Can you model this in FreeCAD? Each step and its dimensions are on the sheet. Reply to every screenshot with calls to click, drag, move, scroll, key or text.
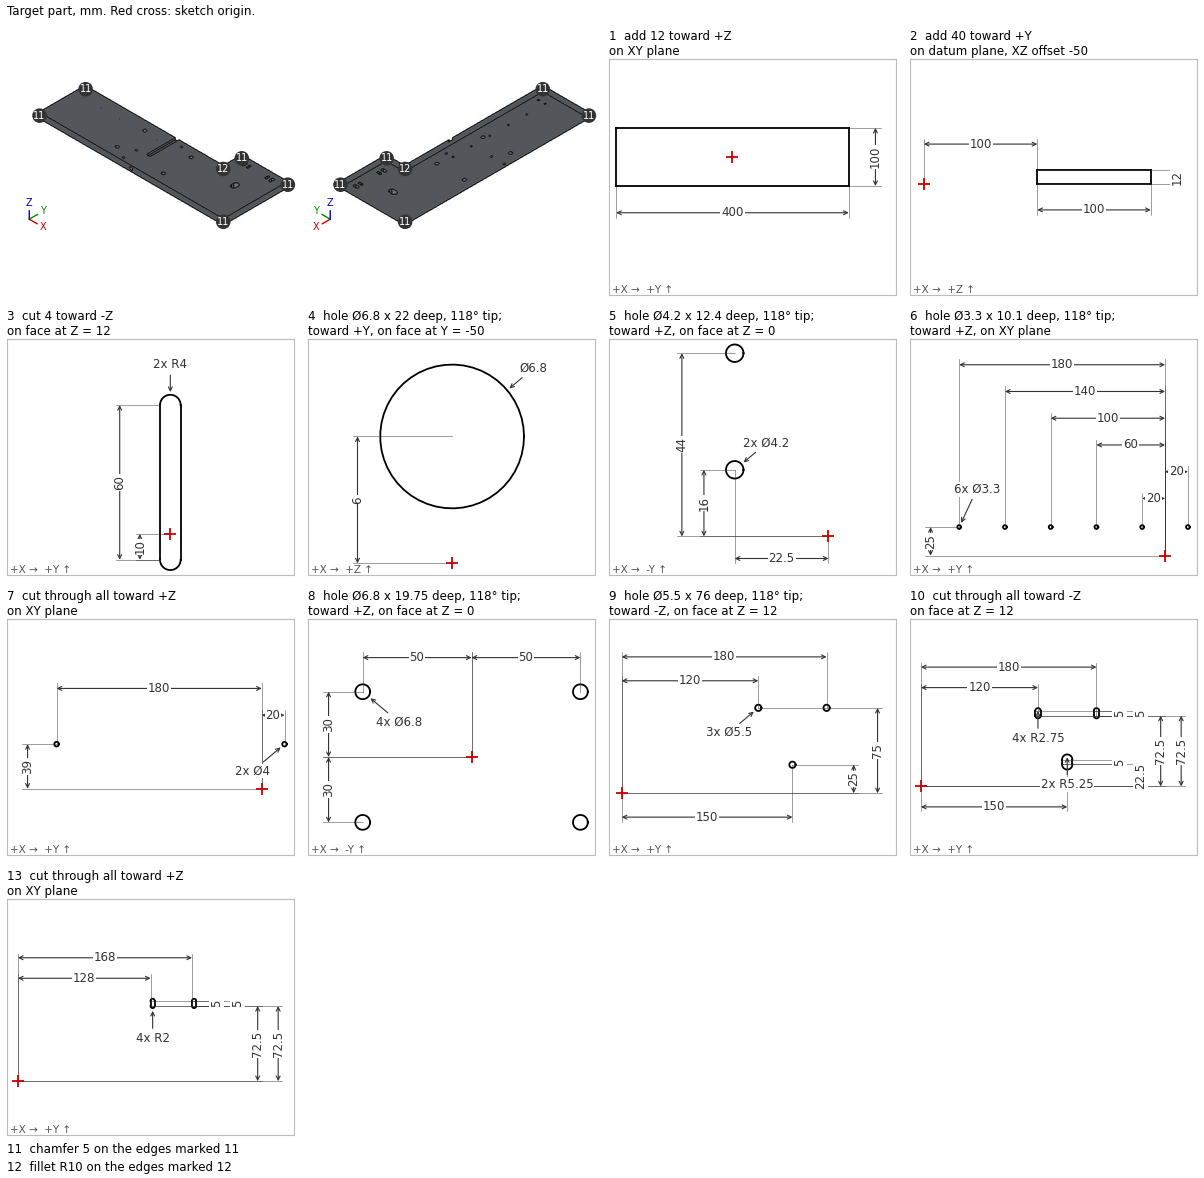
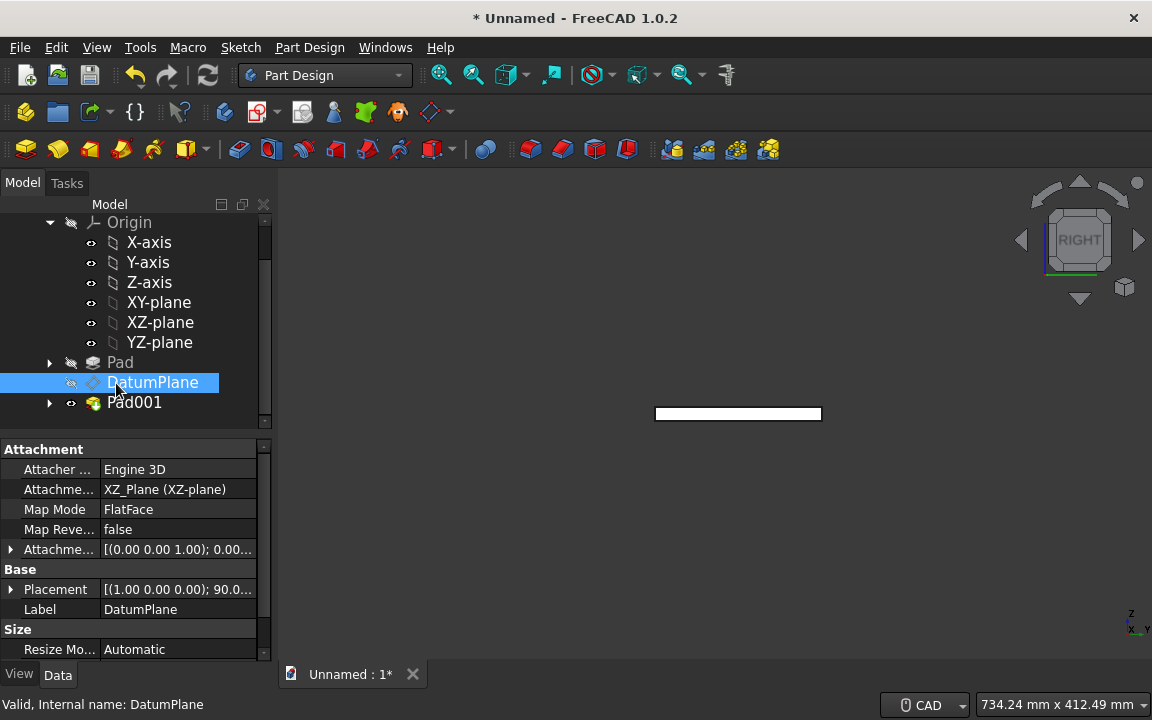
click(442, 76)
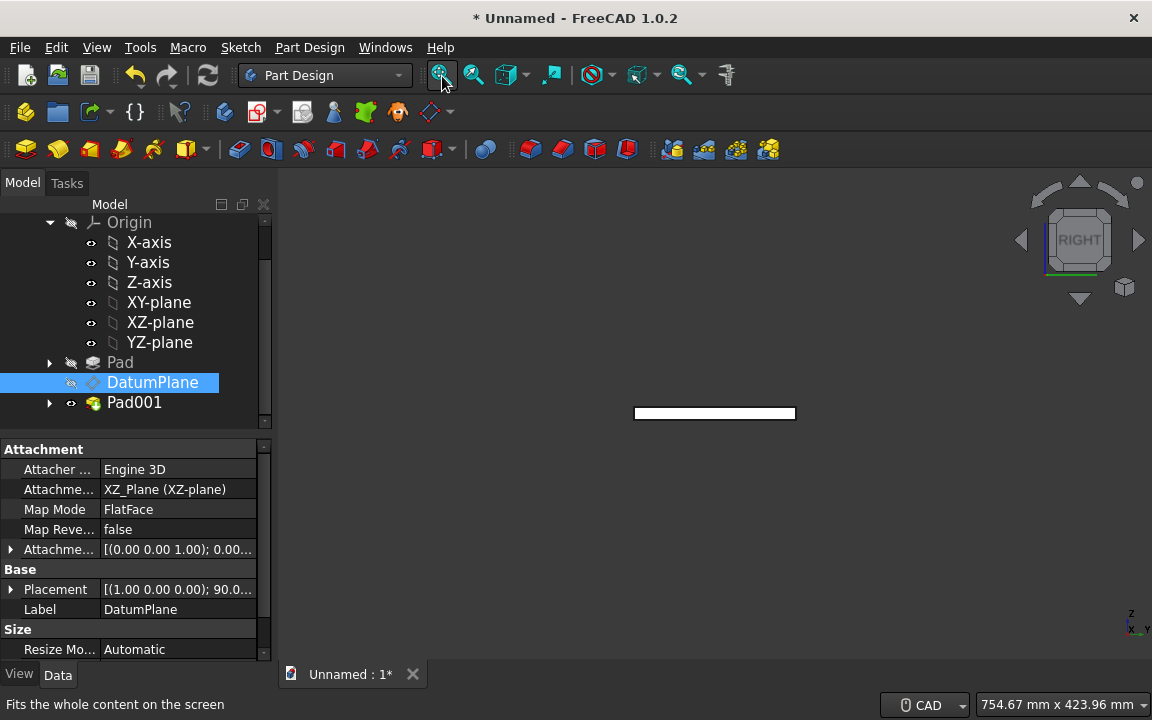
key(0)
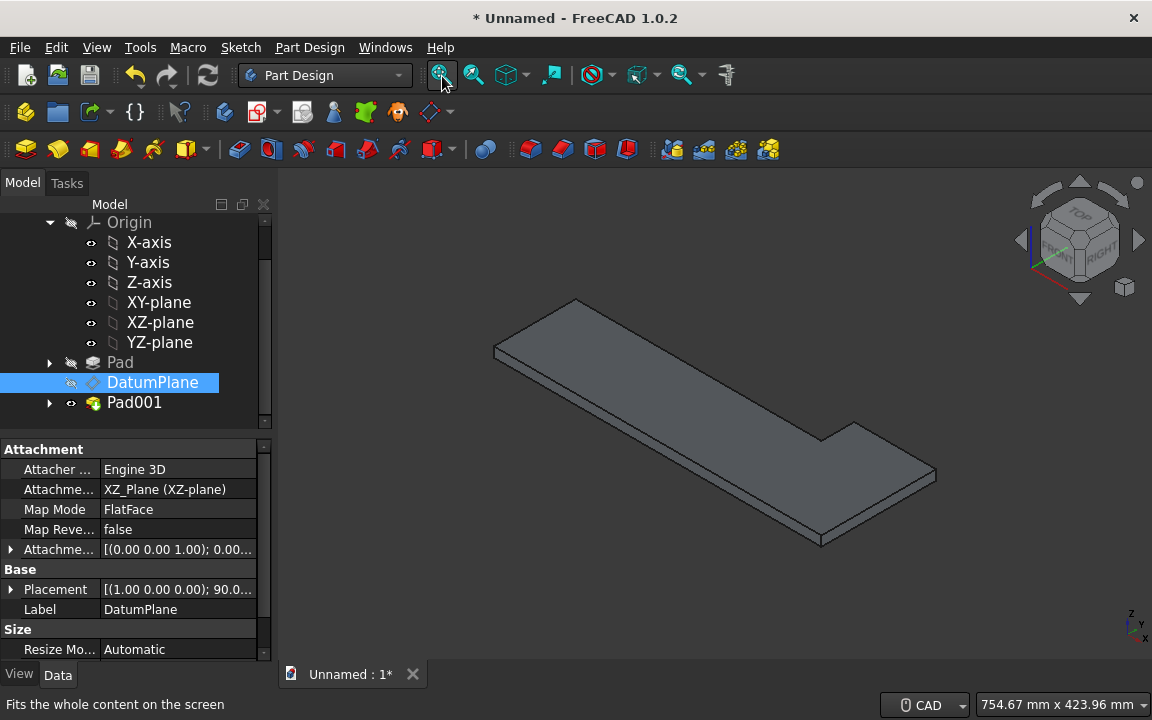
click(792, 470)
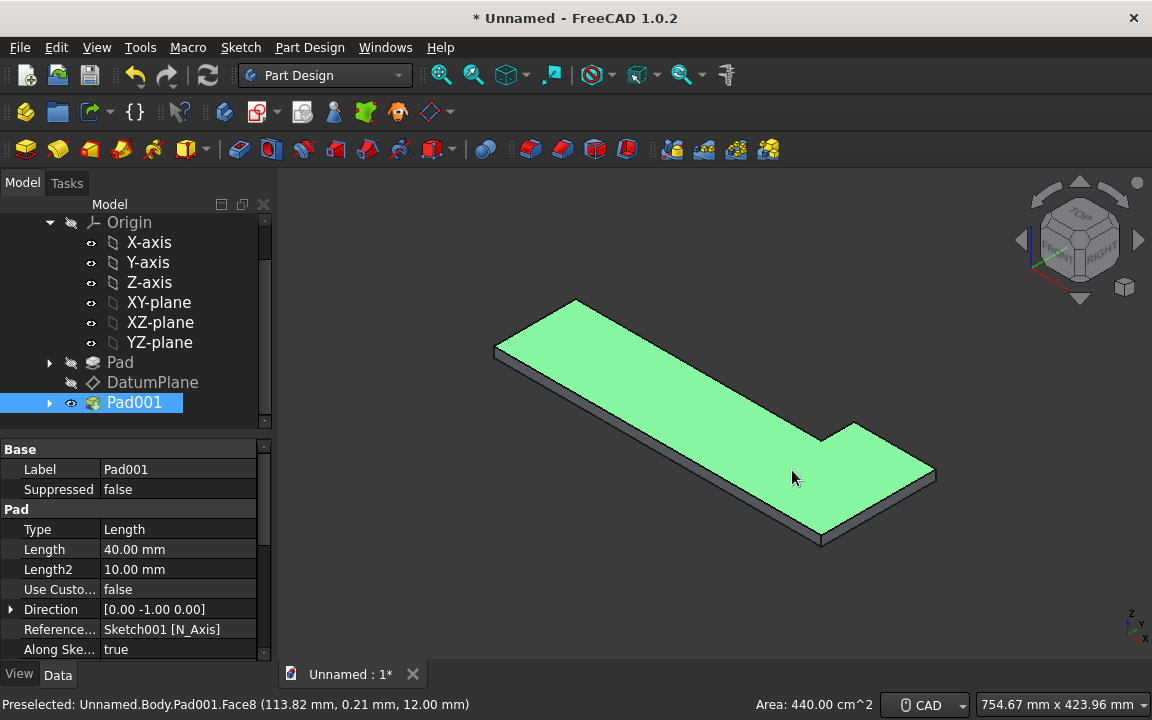
click(258, 112)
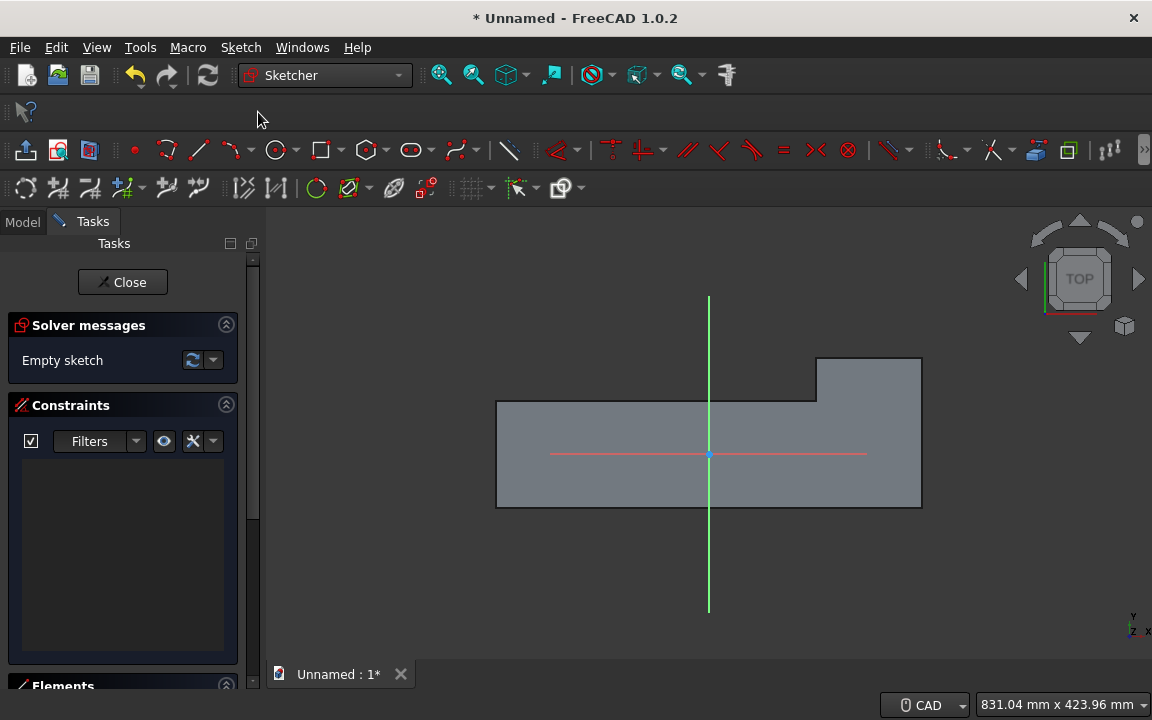
scroll(731, 433, up, 7)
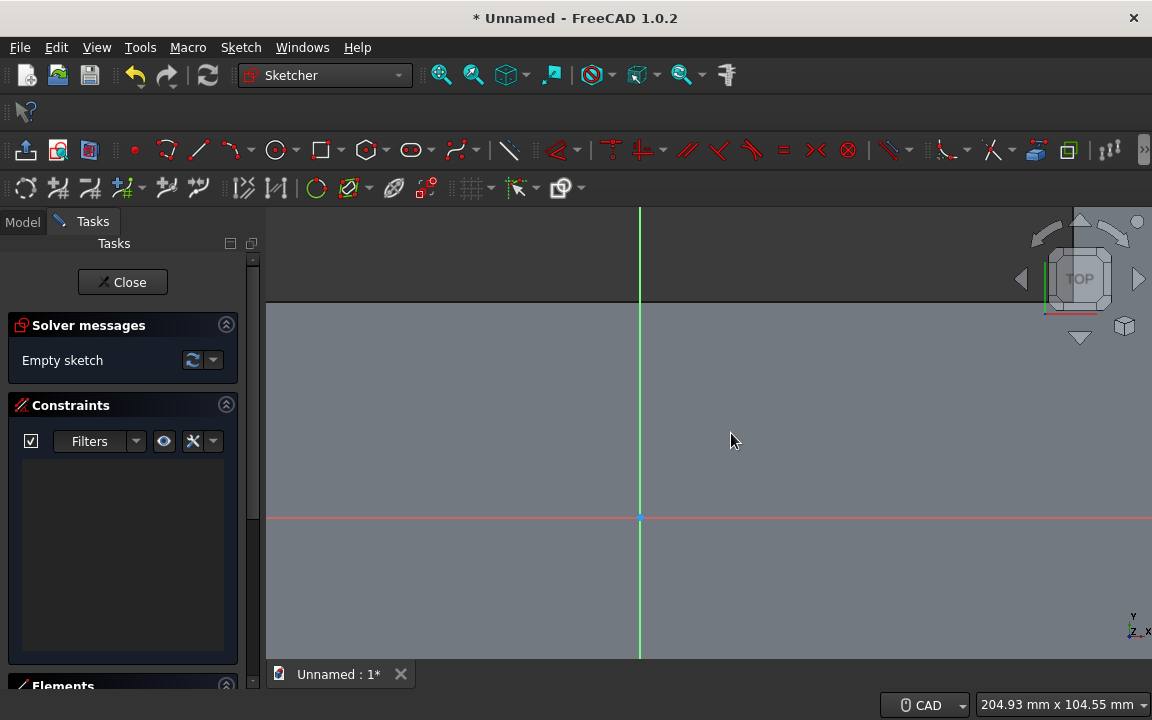
click(412, 150)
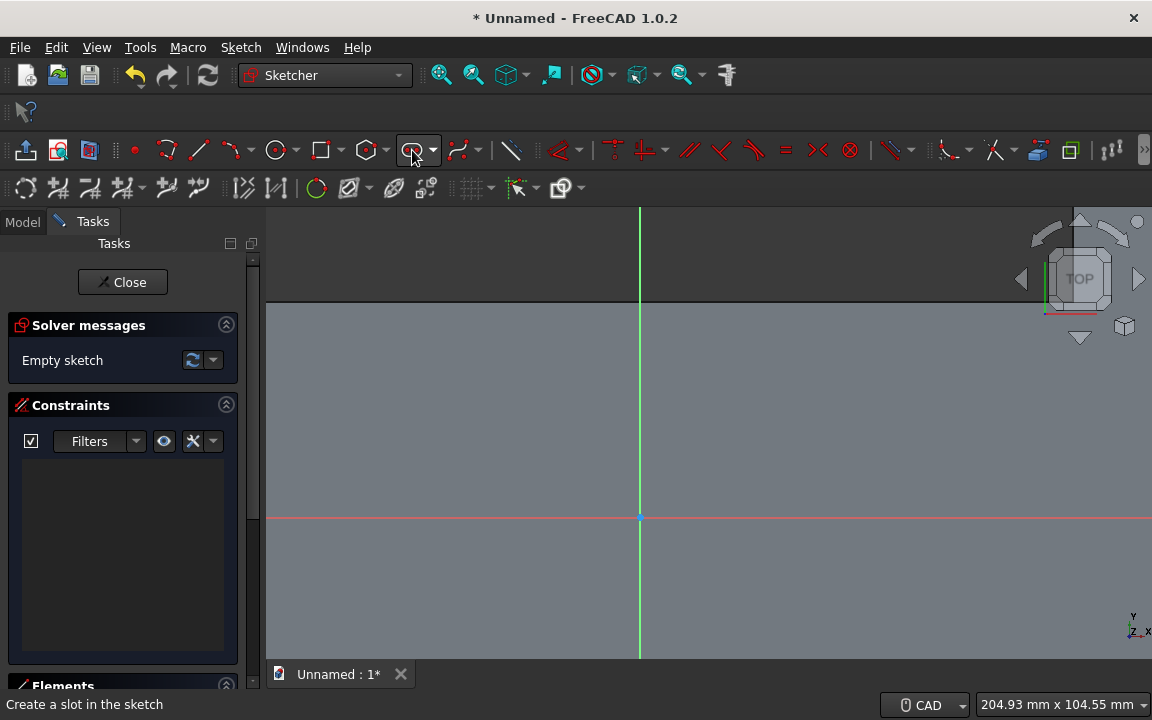
scroll(640, 561, up, 2)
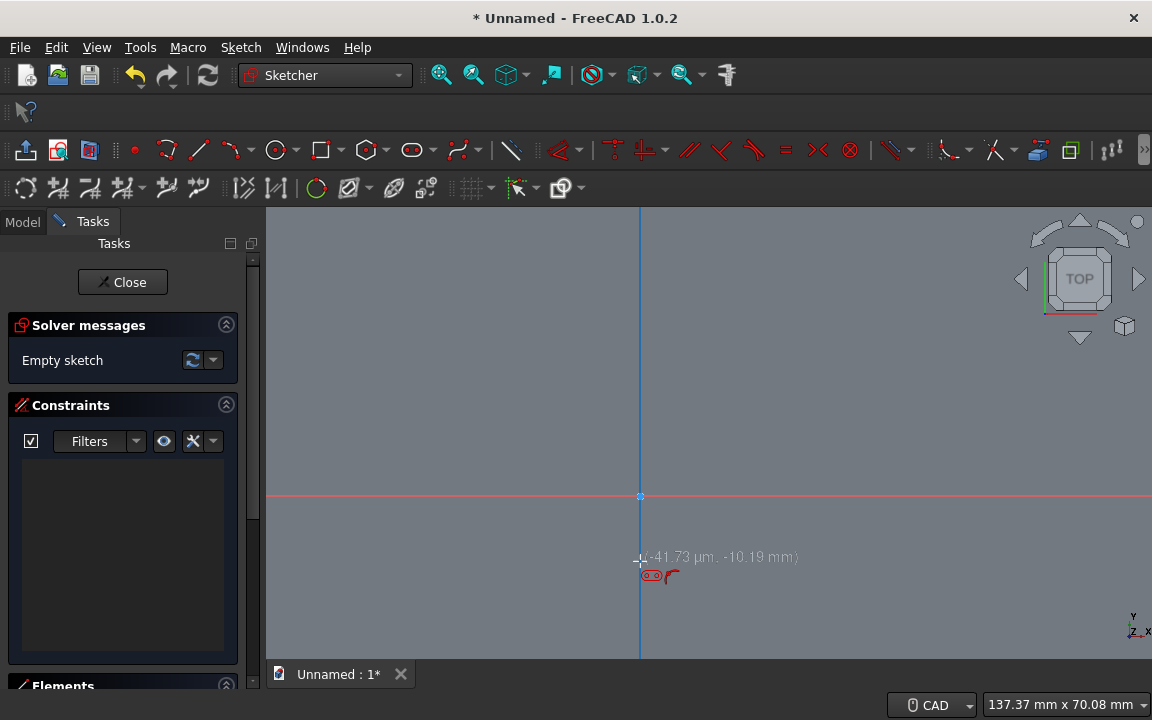
click(640, 561)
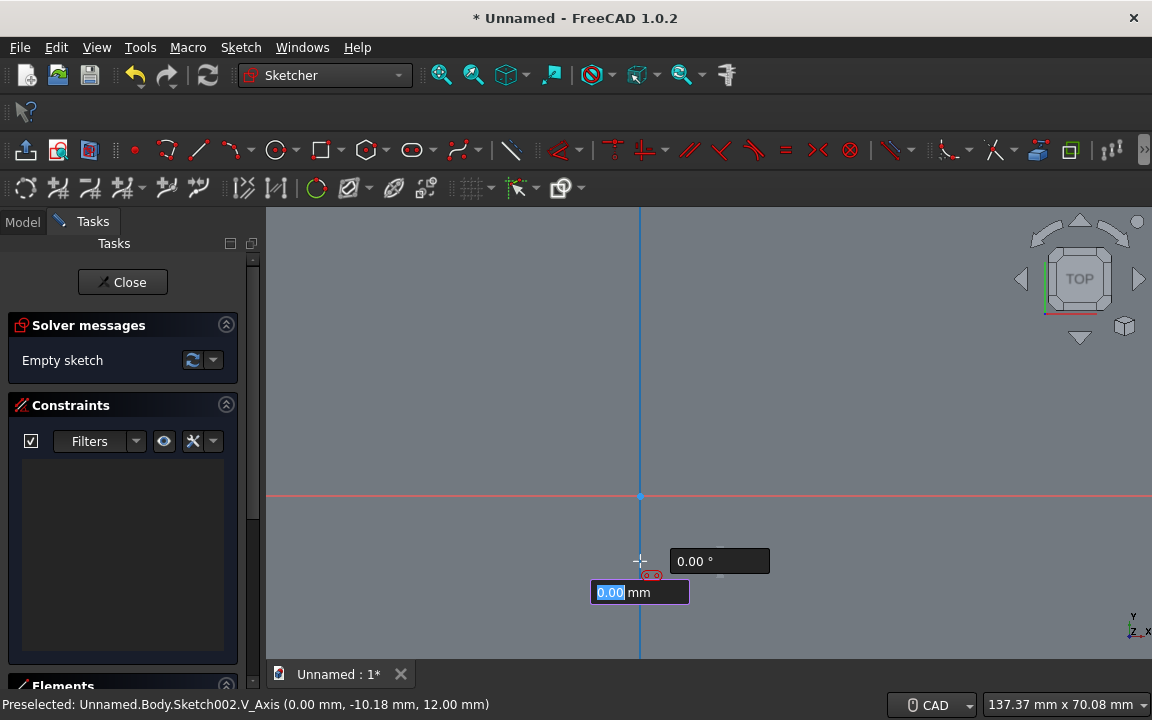
scroll(641, 566, down, 2)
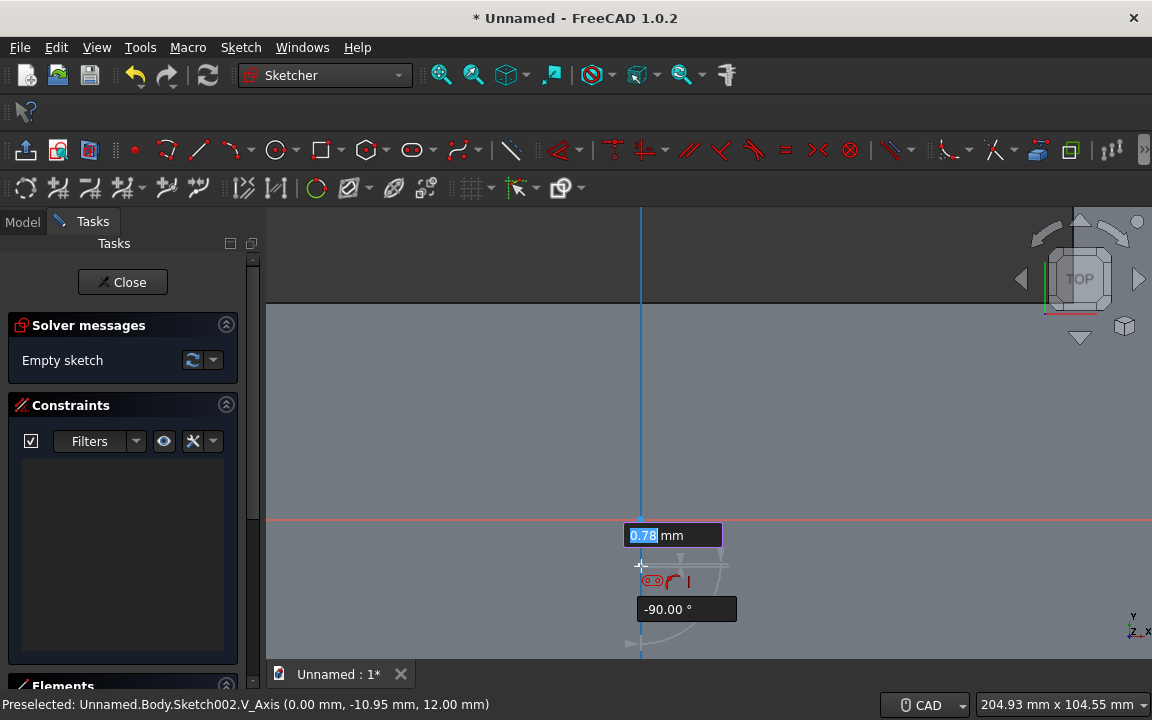
click(650, 303)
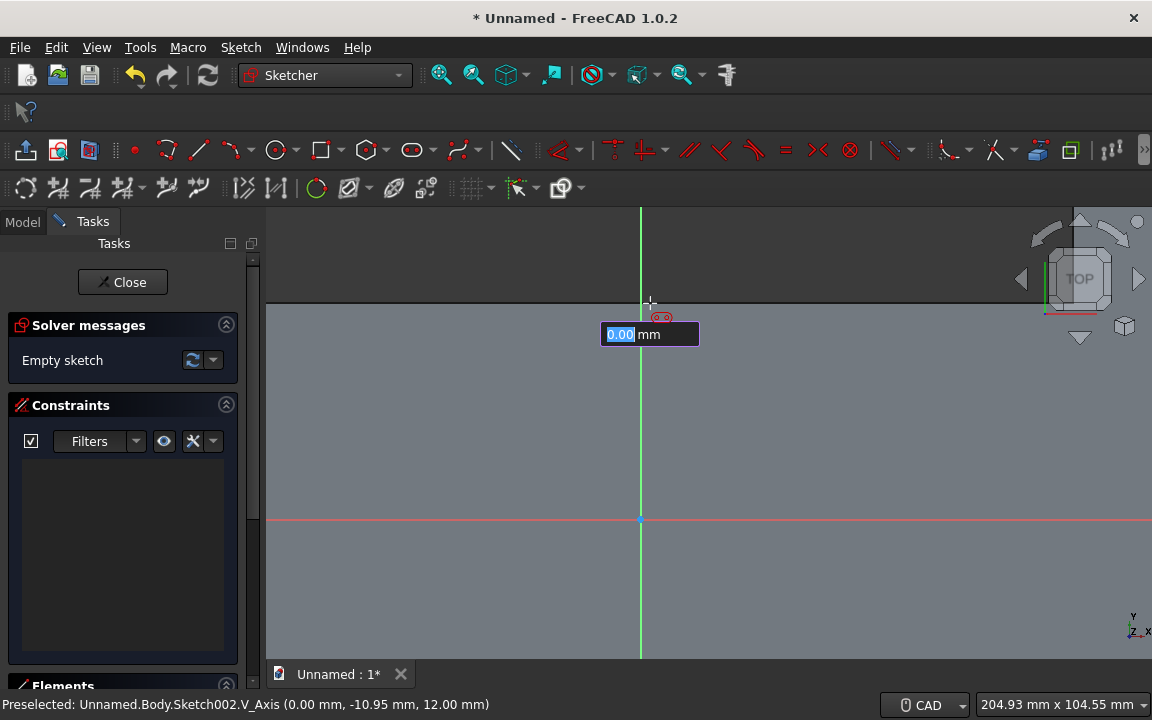
click(658, 433)
key(Escape)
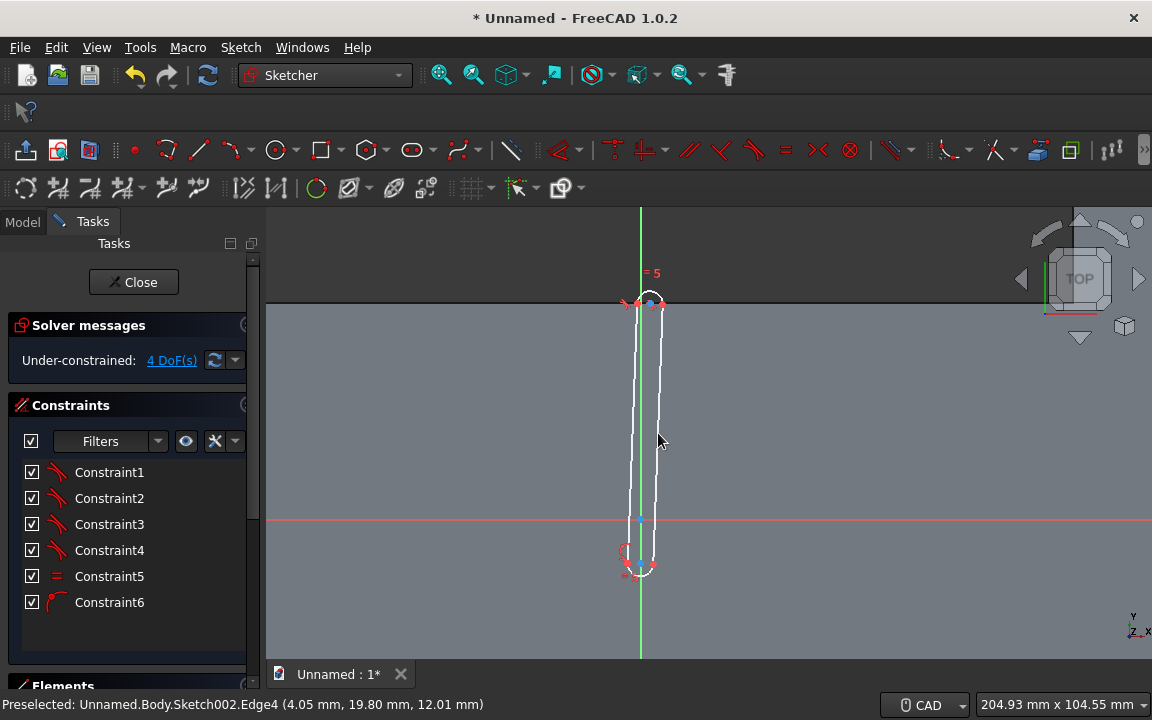
scroll(631, 485, up, 2)